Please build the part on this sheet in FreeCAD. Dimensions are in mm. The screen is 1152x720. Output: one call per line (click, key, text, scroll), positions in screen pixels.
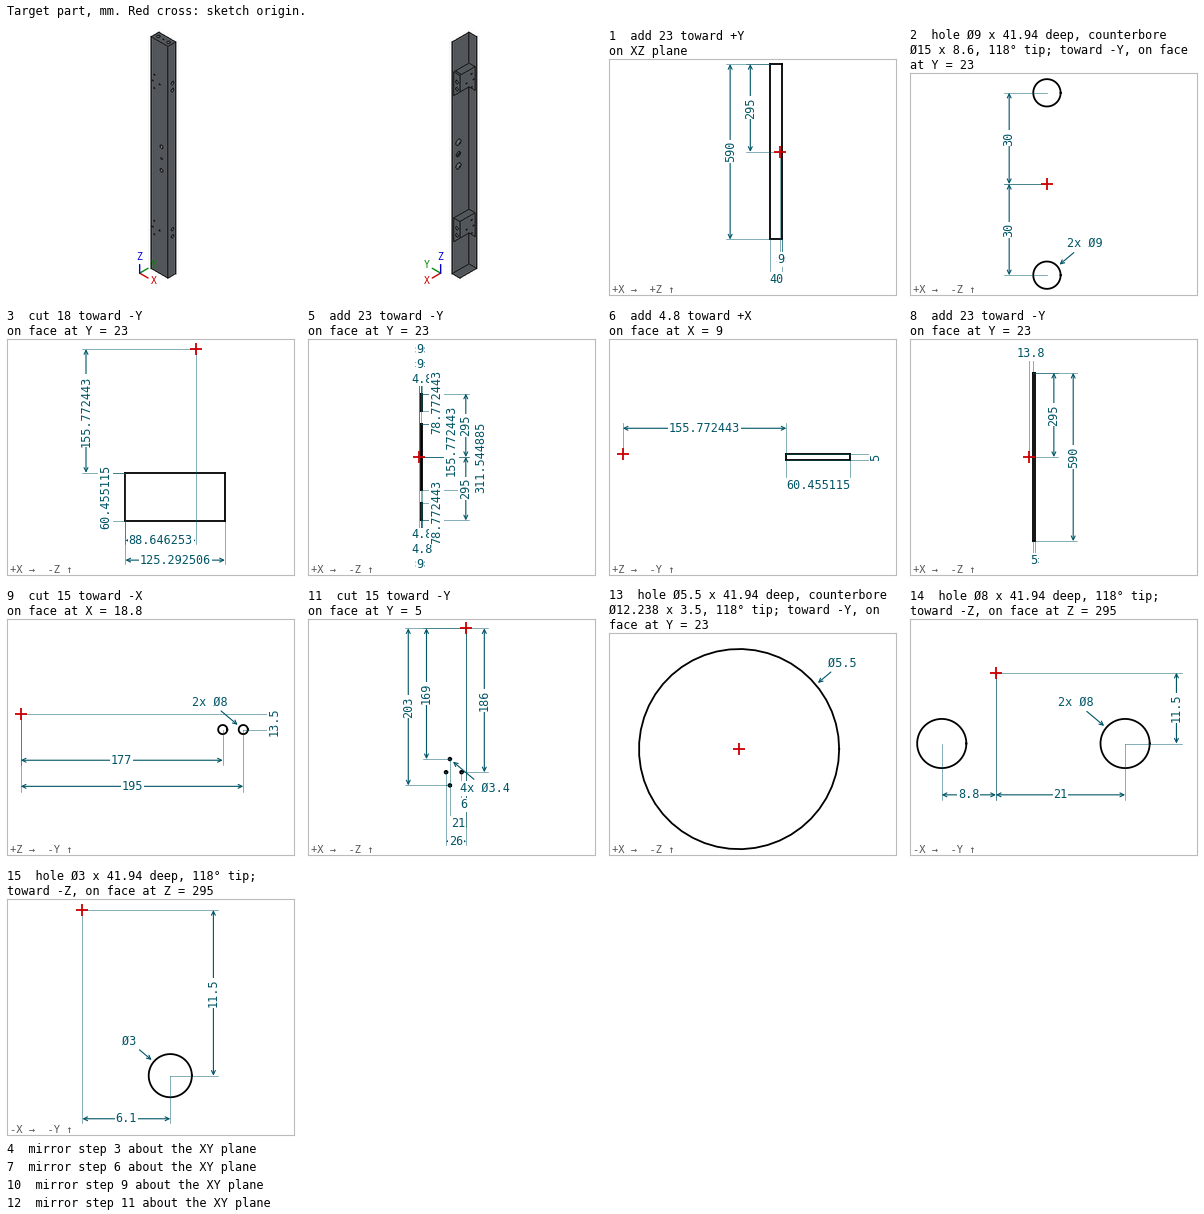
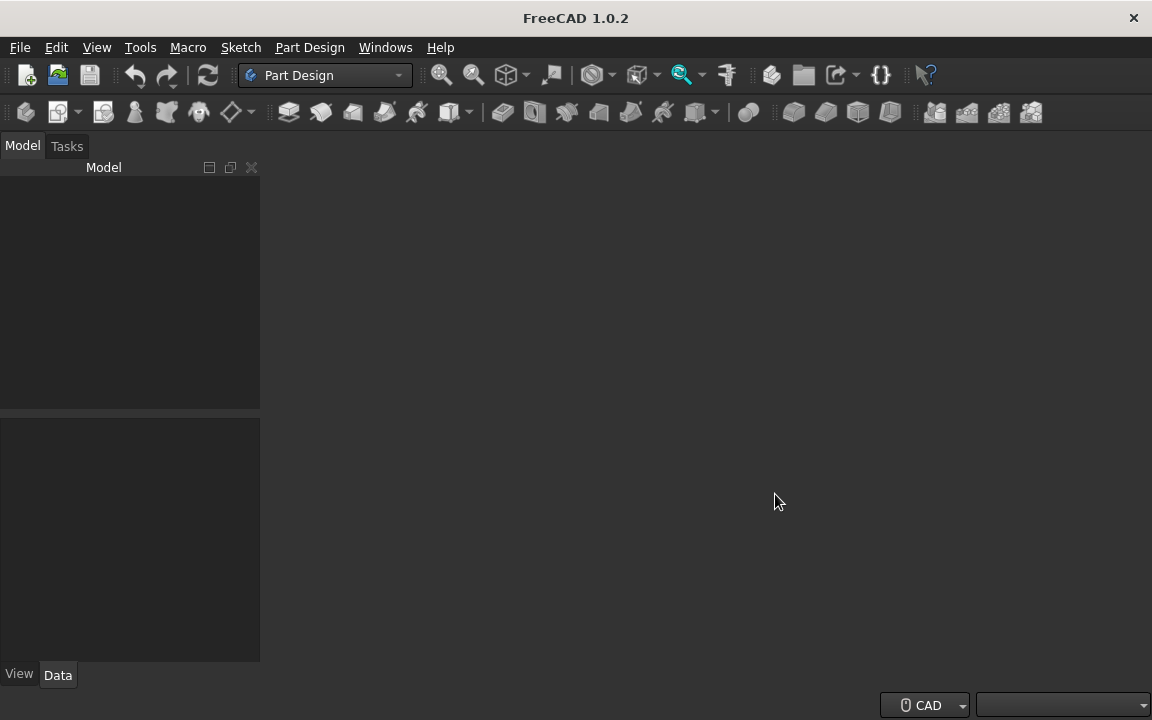
click(26, 76)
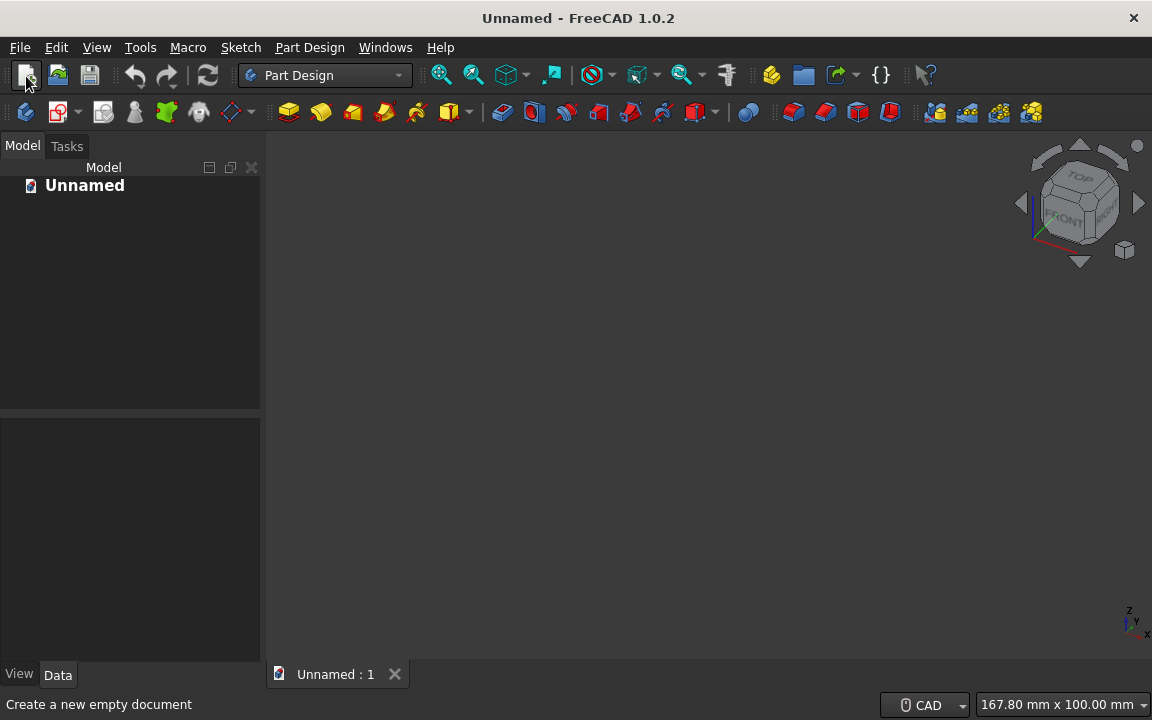
click(58, 112)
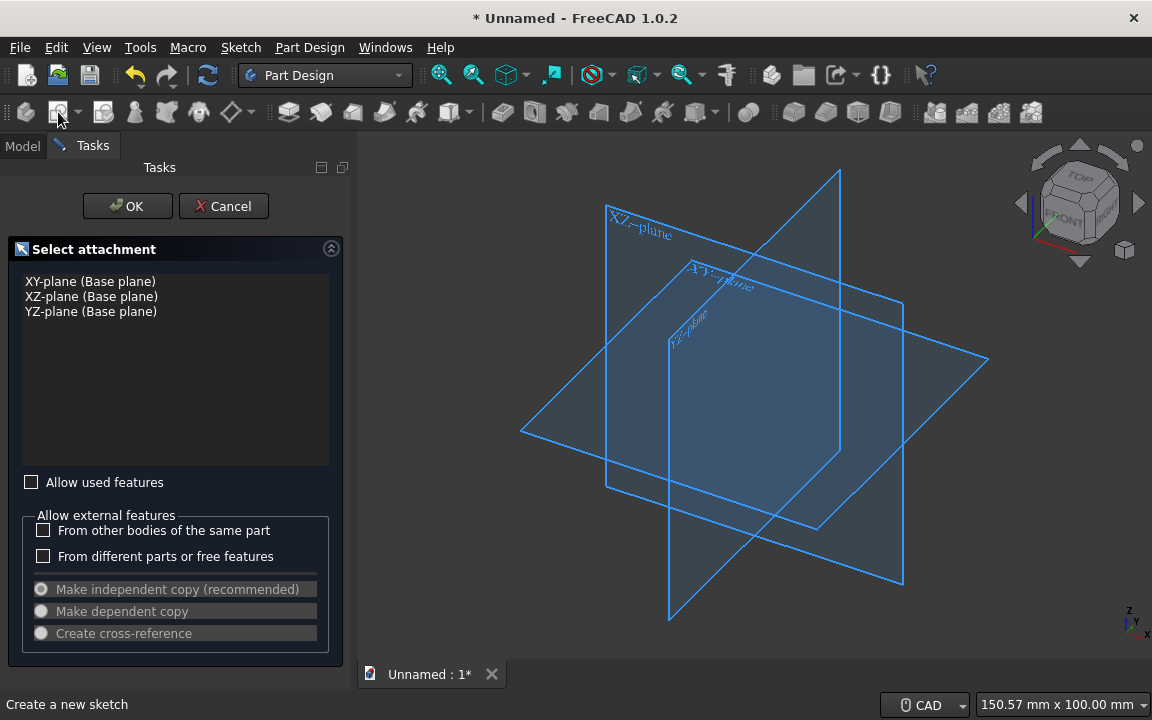
click(82, 296)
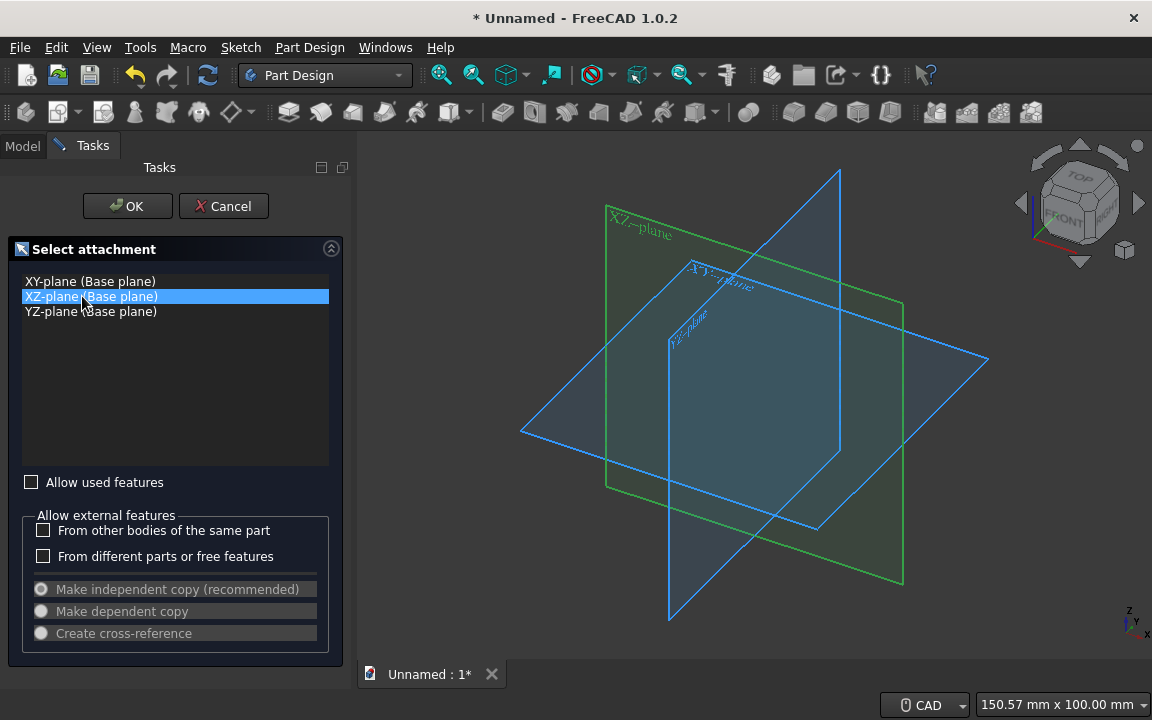
click(128, 206)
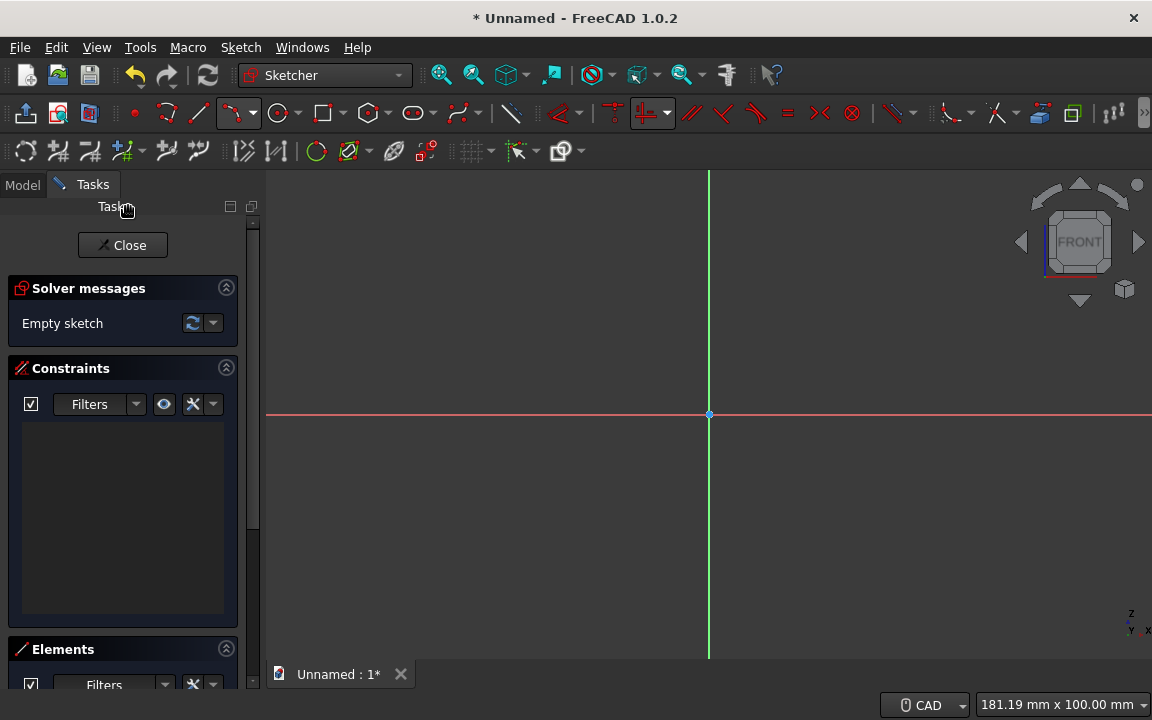
scroll(639, 414, down, 11)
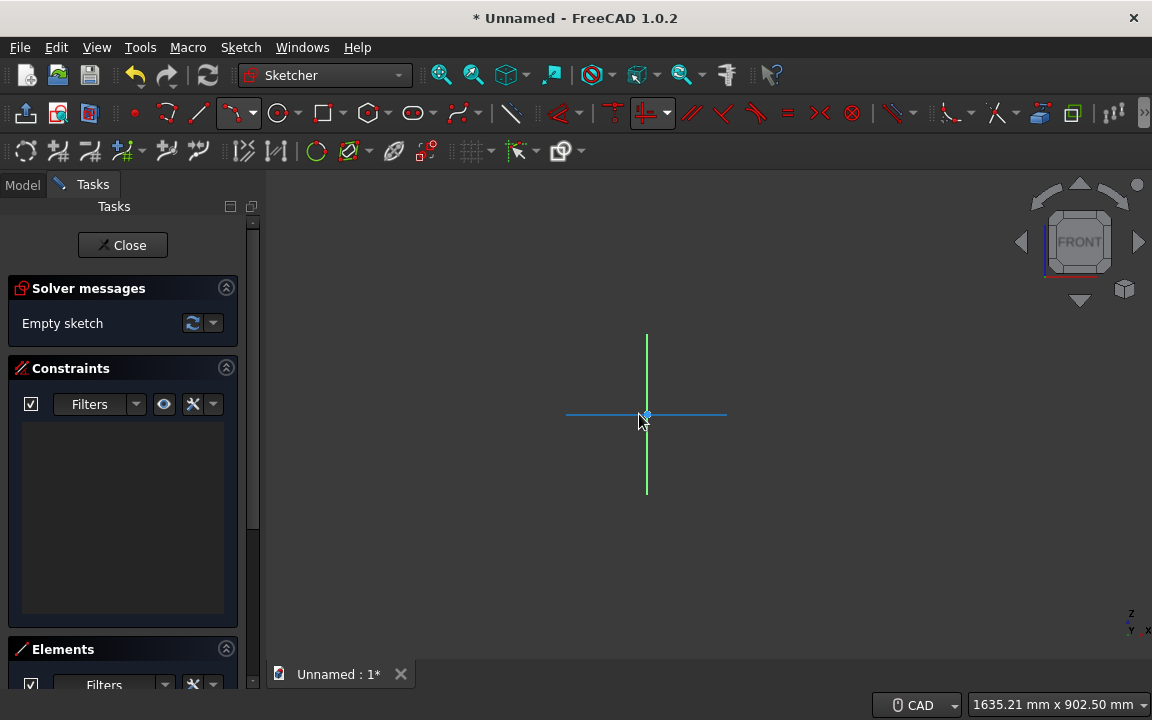
click(324, 114)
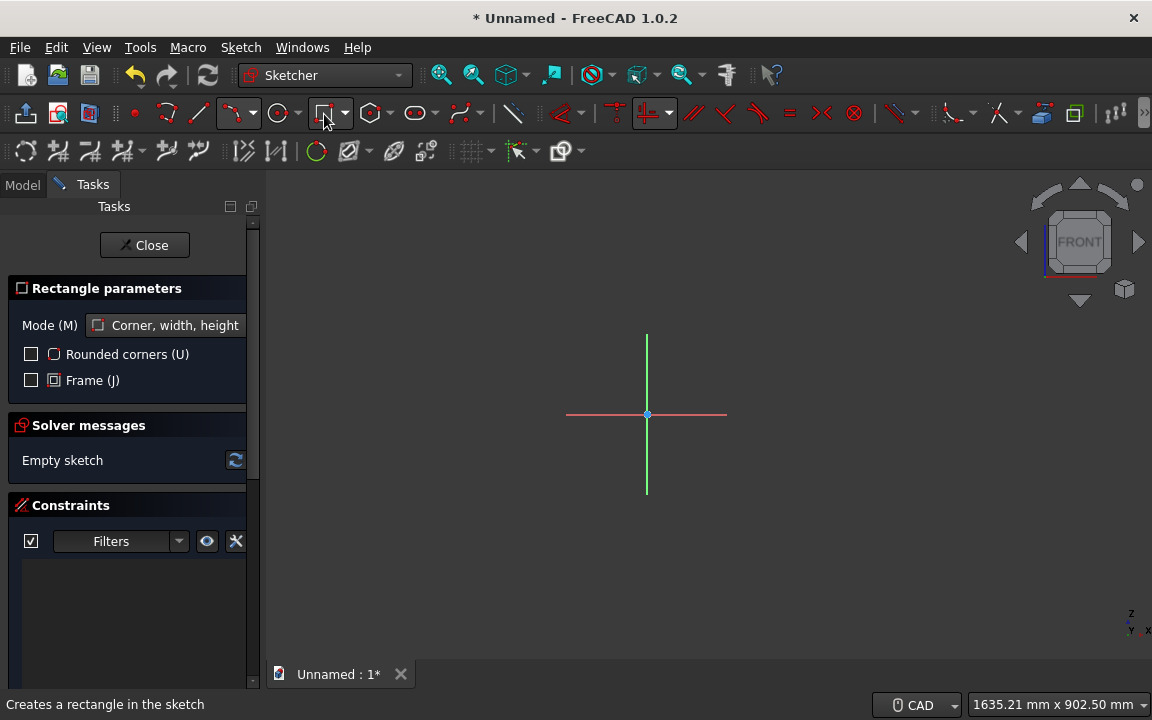
click(630, 255)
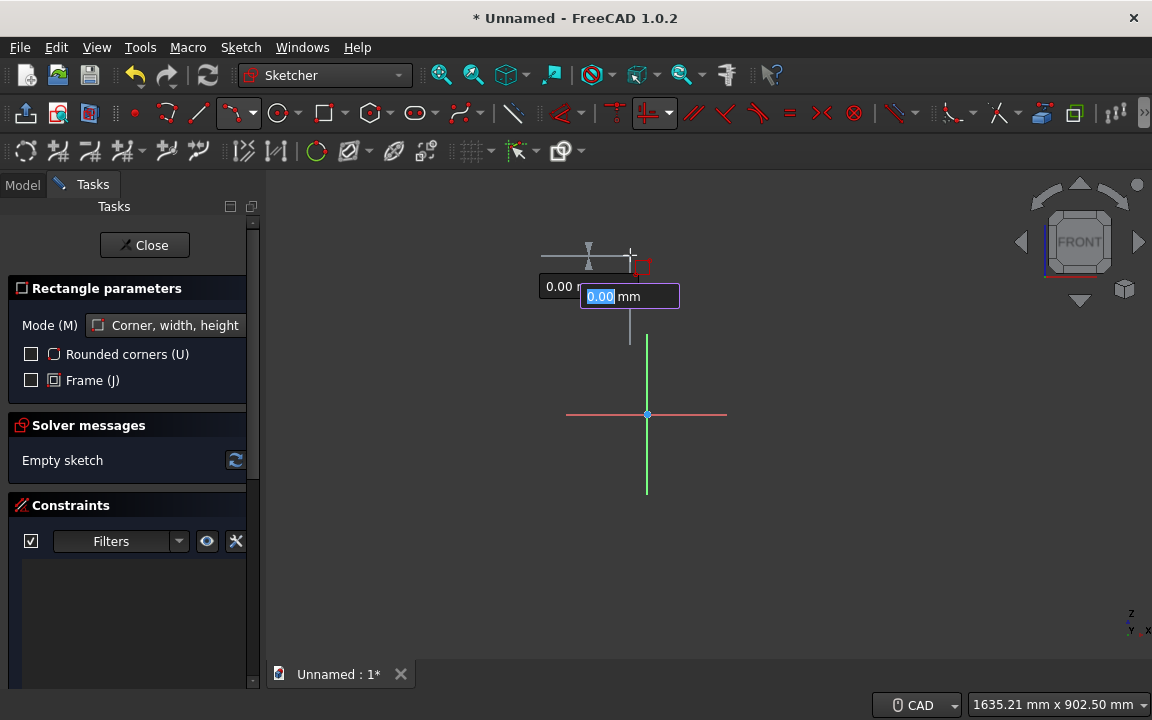
scroll(652, 574, up, 6)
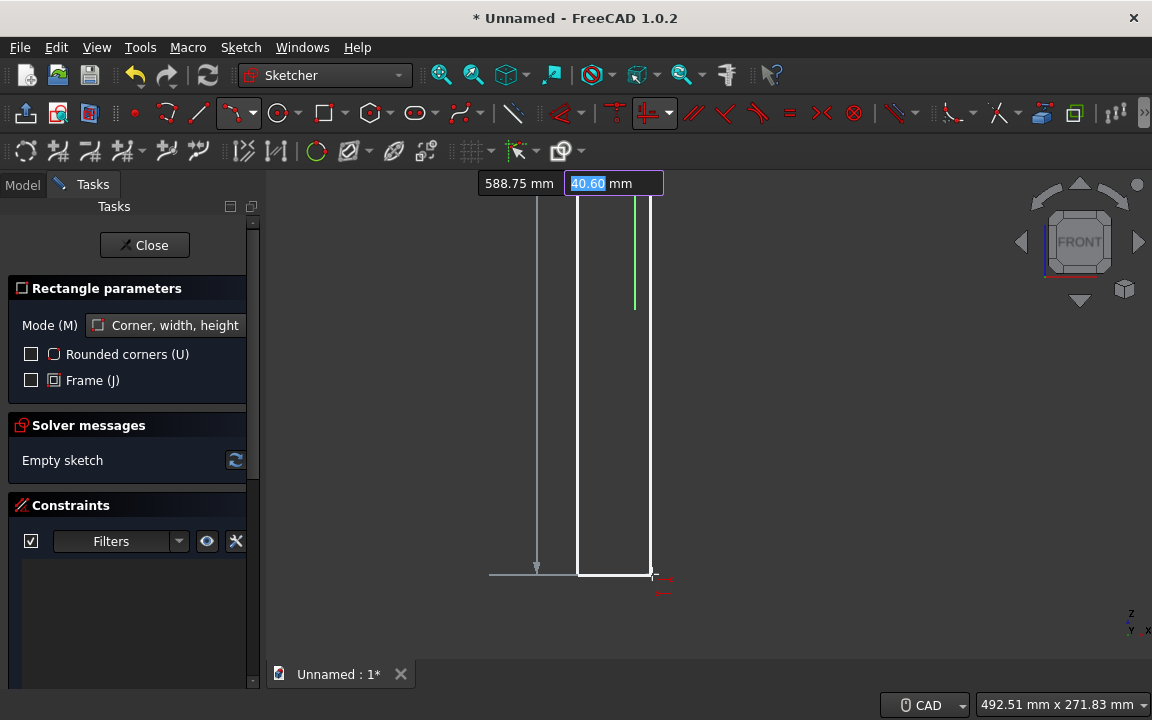
click(651, 573)
key(Escape)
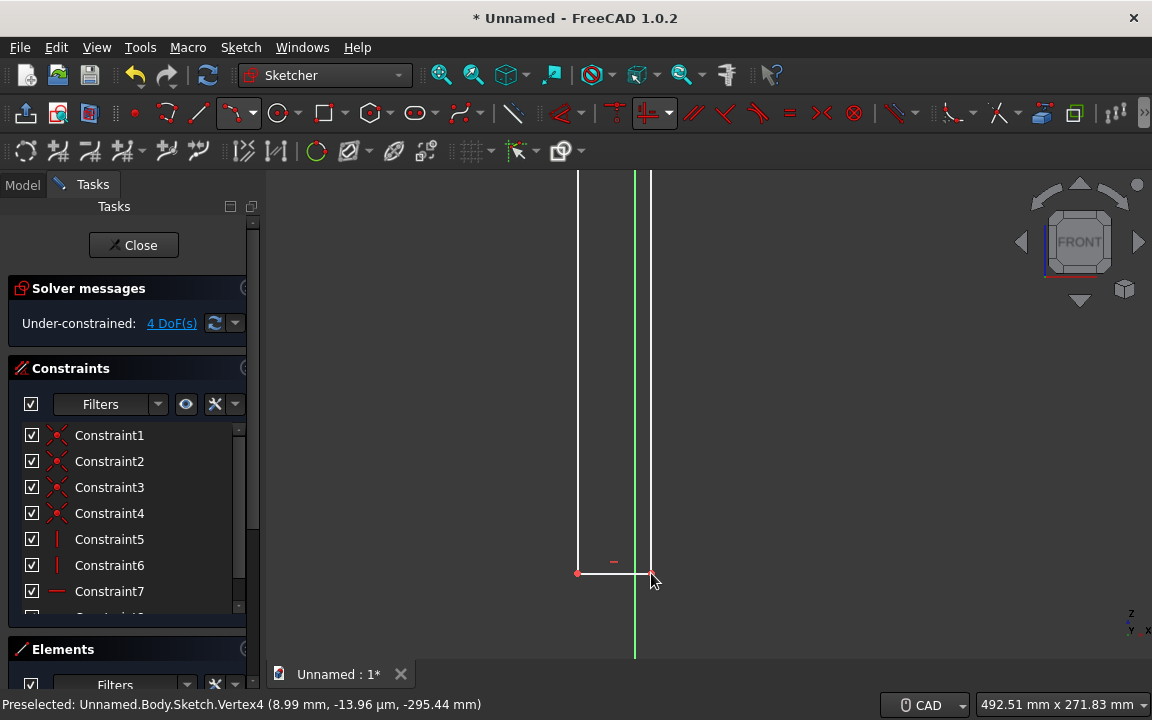
click(560, 114)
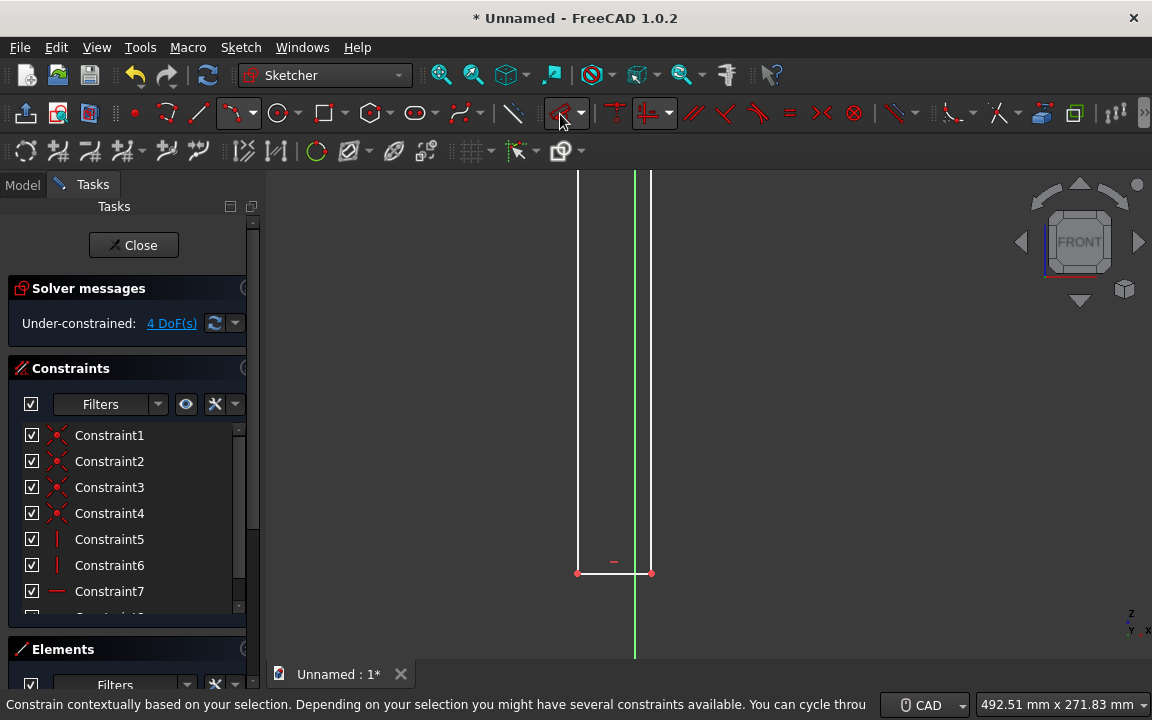
click(600, 574)
click(614, 608)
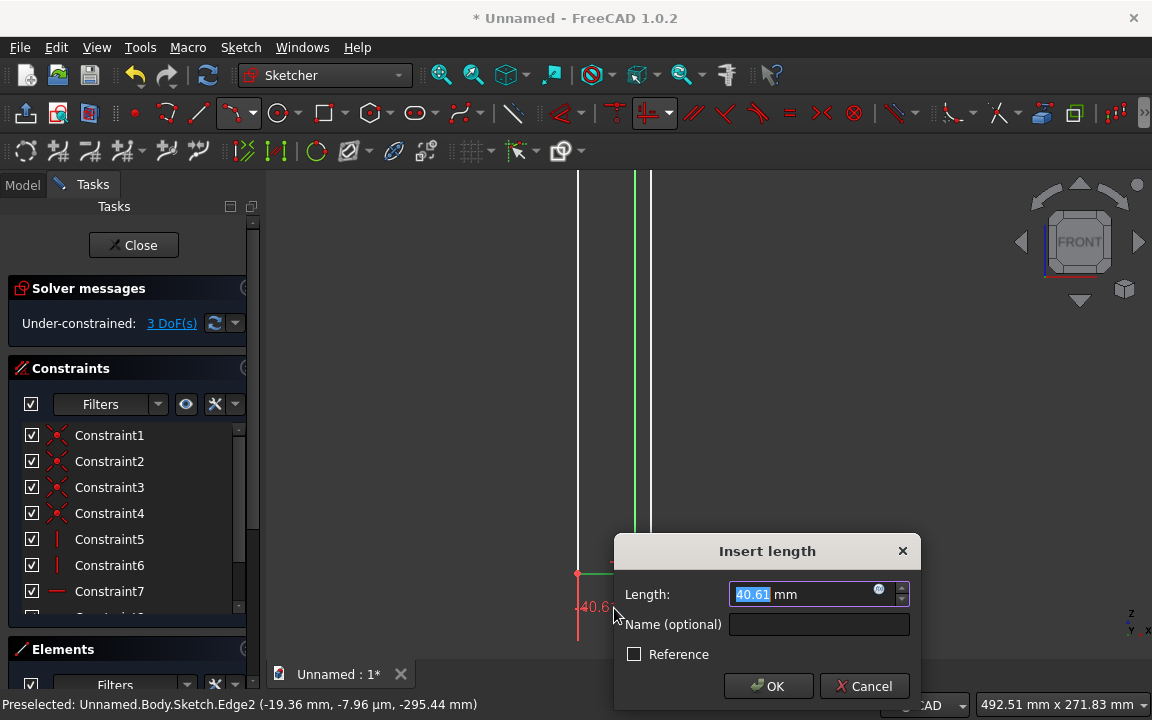
text(40)
key(Return)